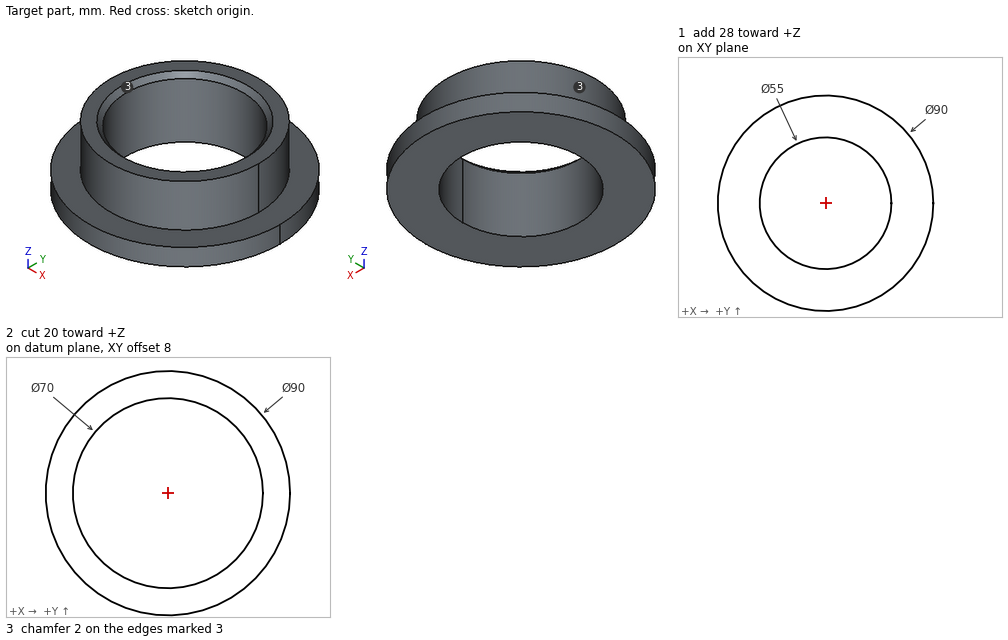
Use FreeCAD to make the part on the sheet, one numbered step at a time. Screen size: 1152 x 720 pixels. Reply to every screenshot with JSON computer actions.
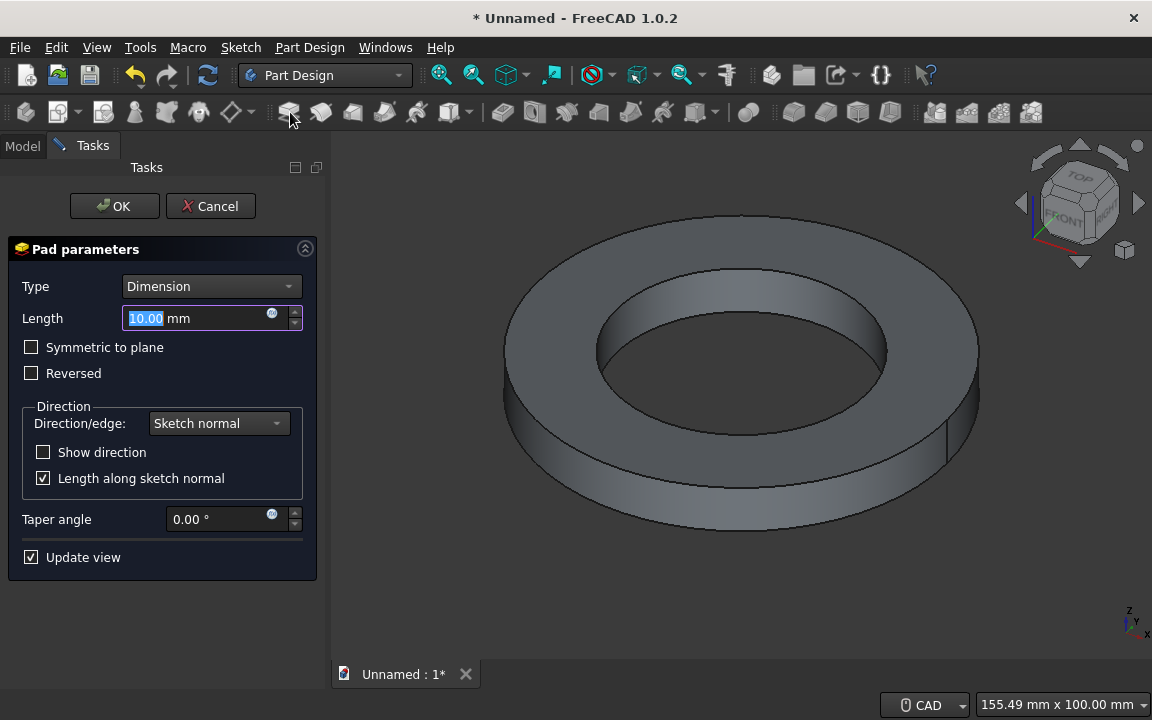
{"action": "type", "text": "28"}
{"action": "key", "text": "Tab"}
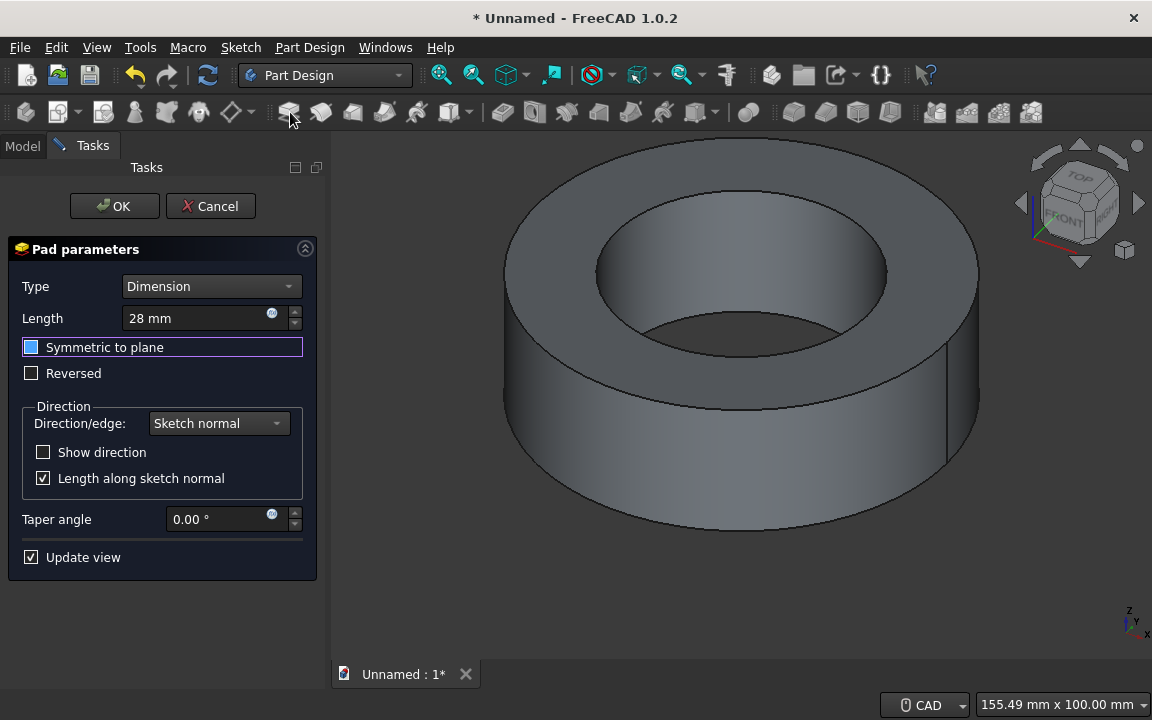
{"action": "left_click", "coordinate": [115, 206]}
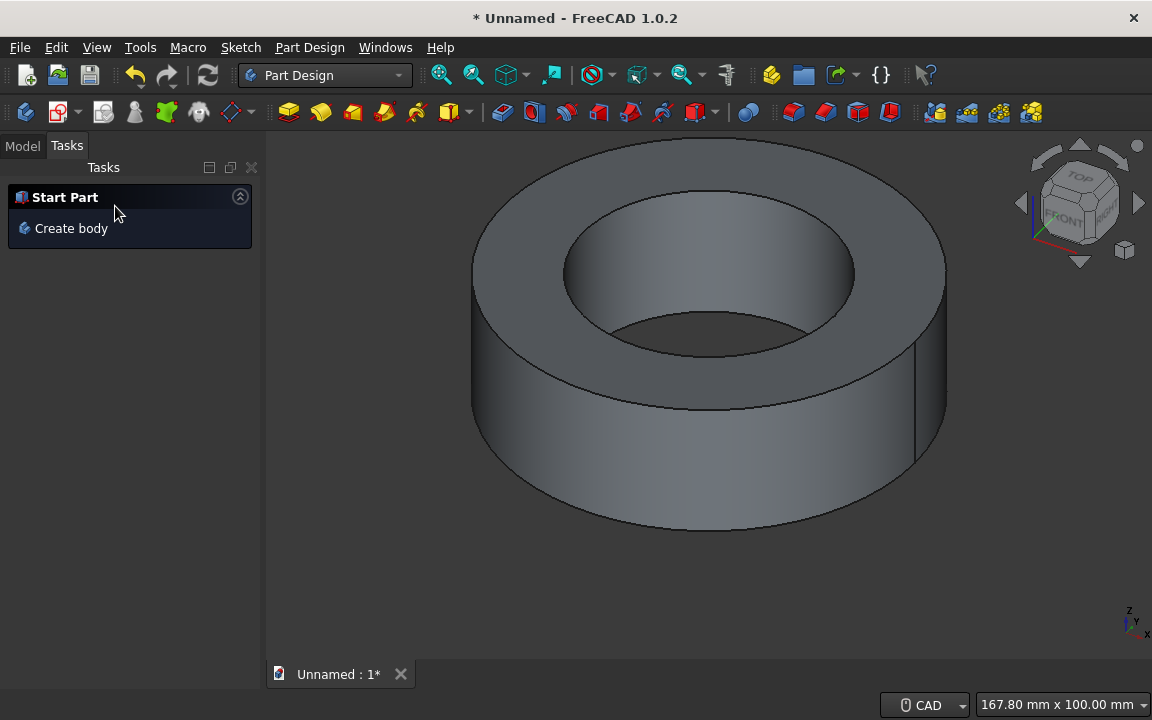
{"action": "left_click", "coordinate": [442, 76]}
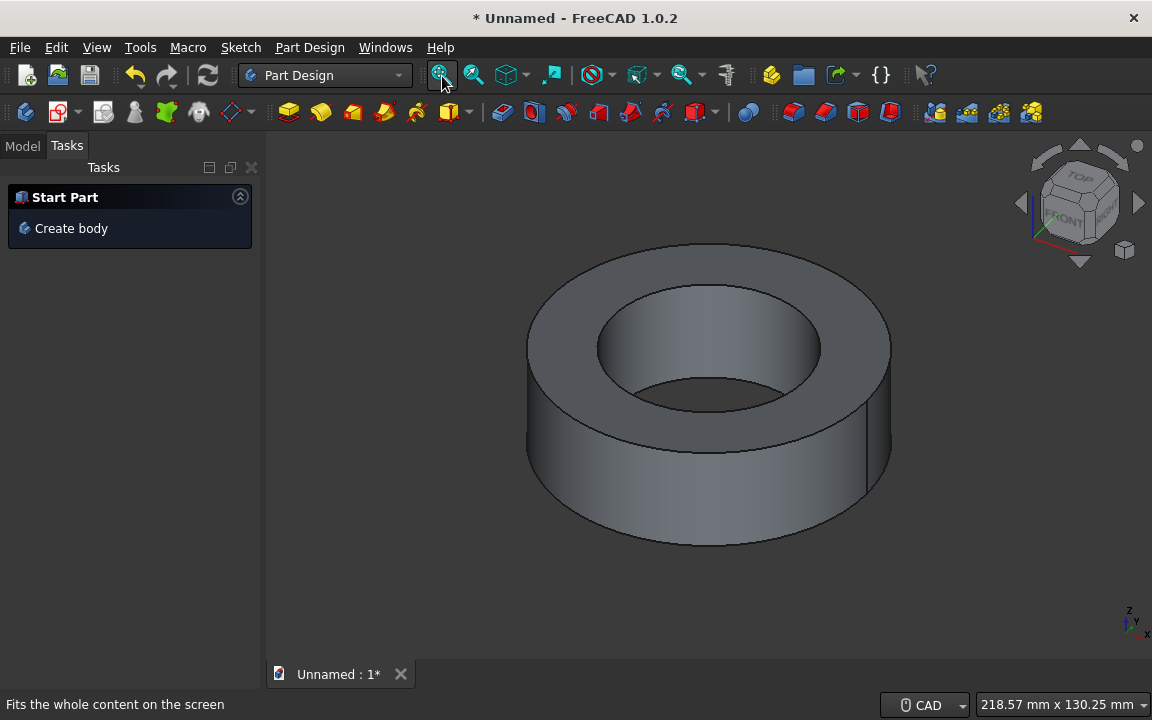
{"action": "left_click", "coordinate": [23, 145]}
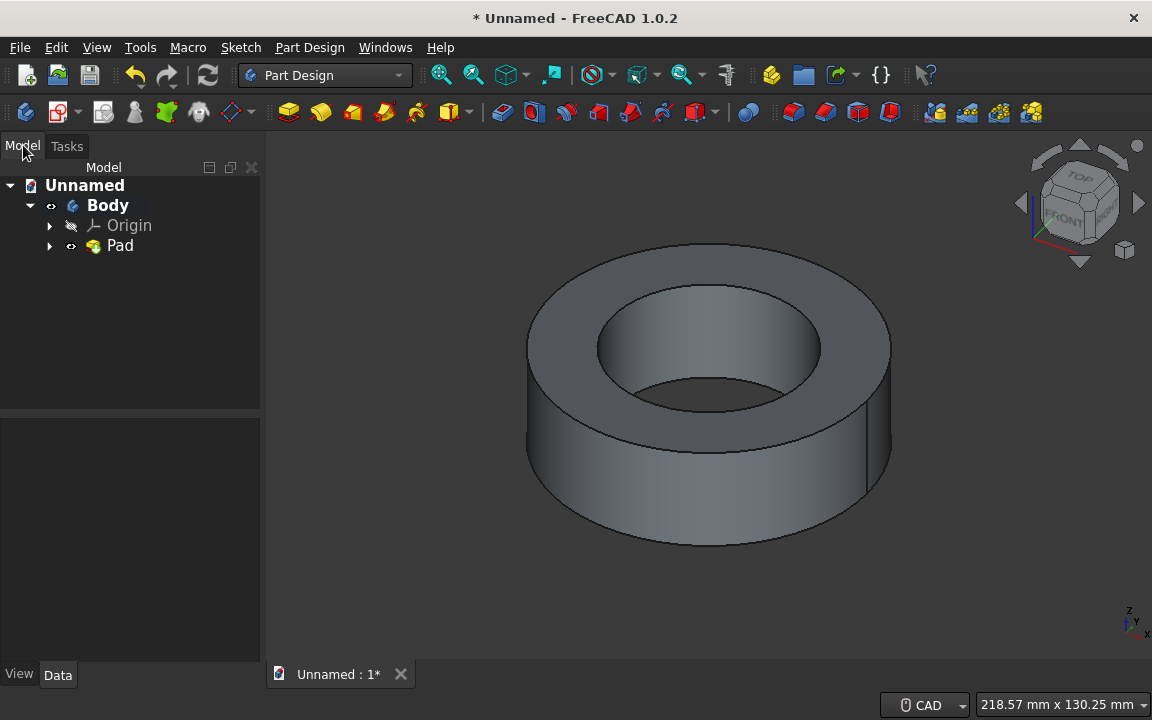
{"action": "left_click", "coordinate": [50, 226]}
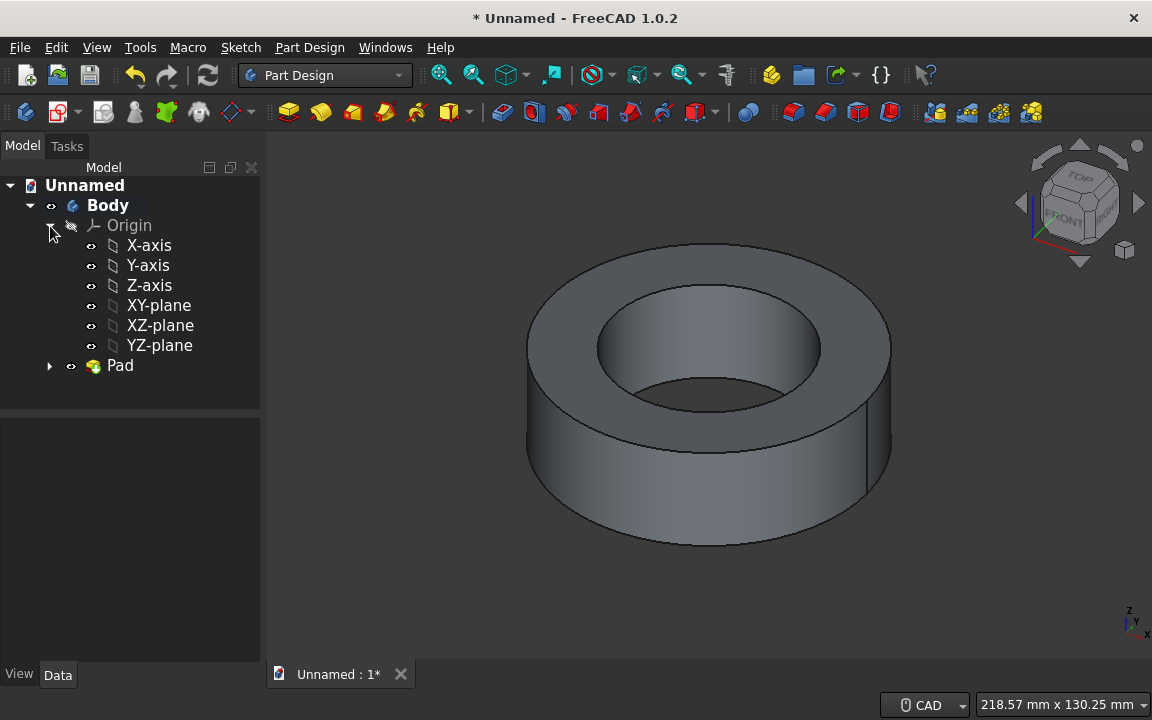
{"action": "left_click", "coordinate": [136, 306]}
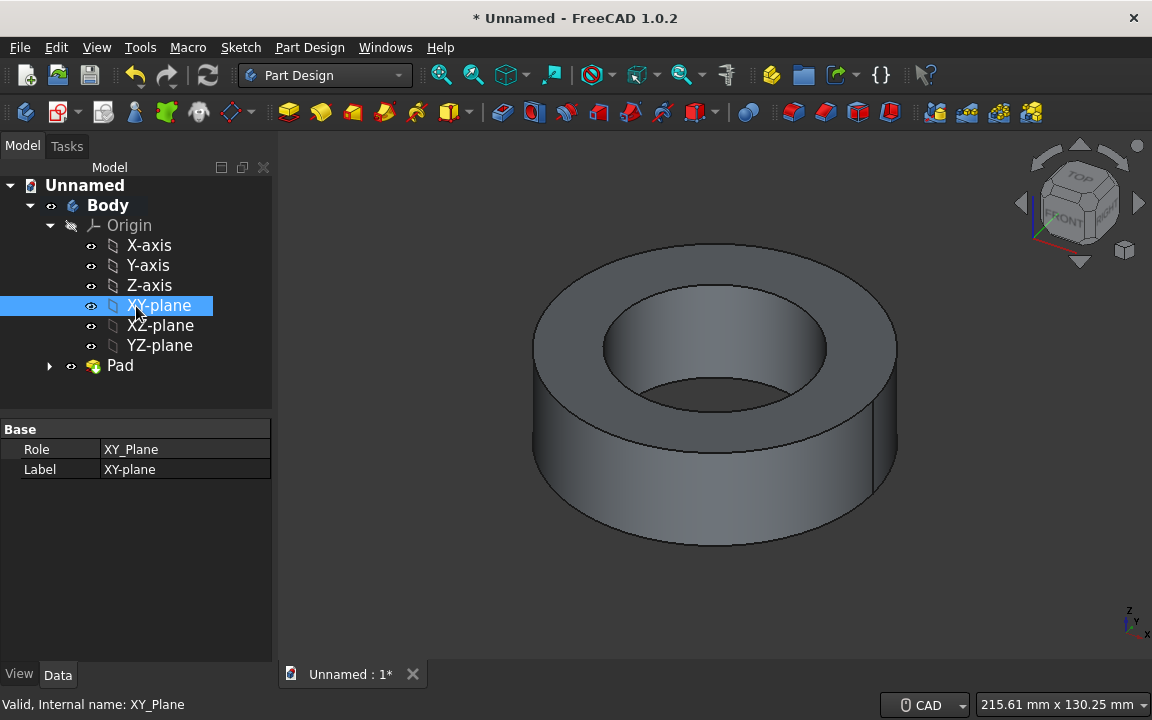
{"action": "left_click", "coordinate": [232, 112]}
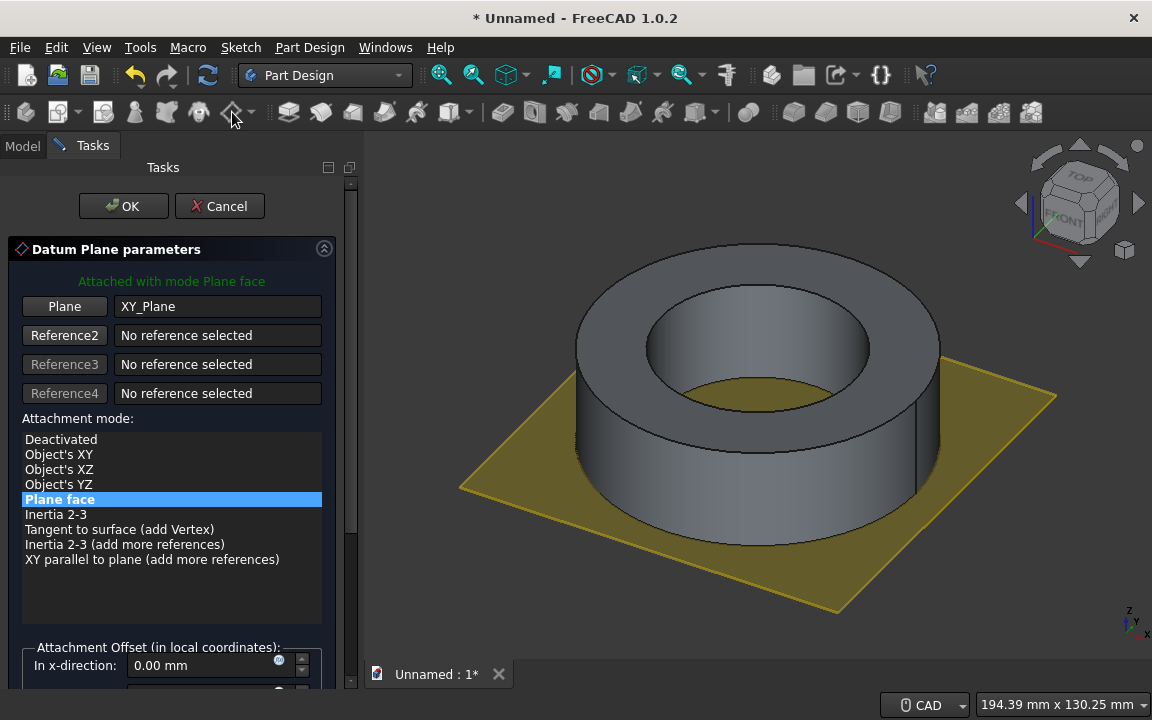
{"action": "scroll", "coordinate": [351, 432], "scroll_direction": "down", "scroll_amount": 2}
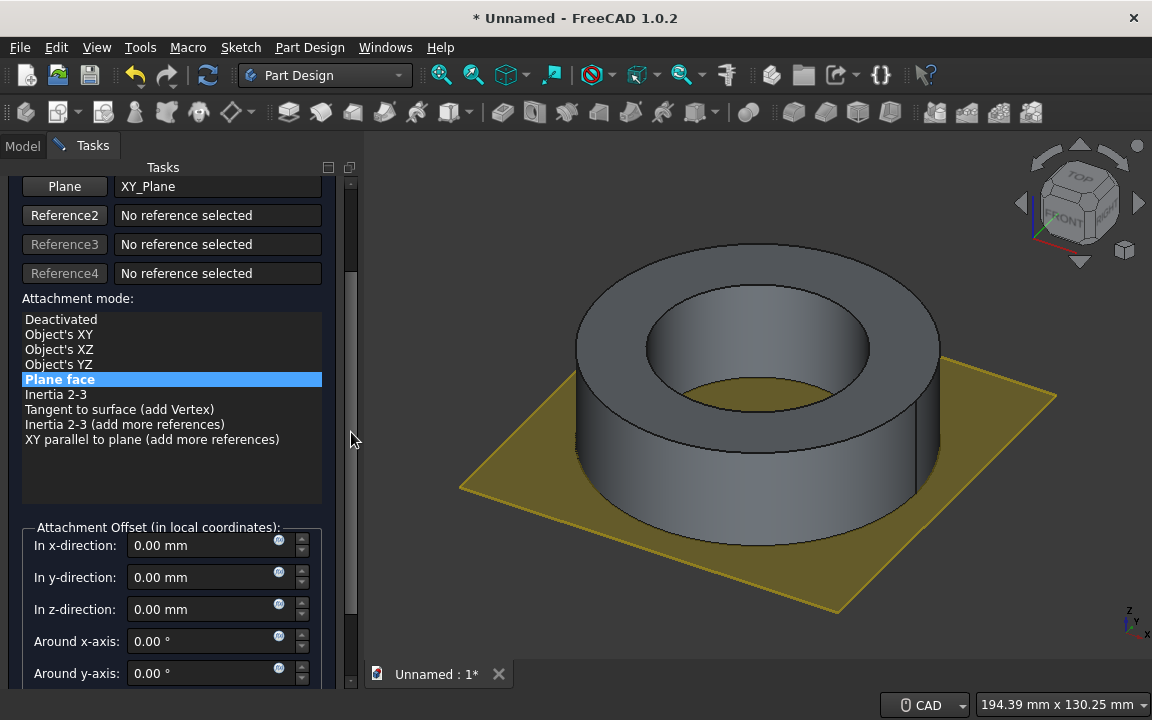
{"action": "triple_click", "coordinate": [210, 609]}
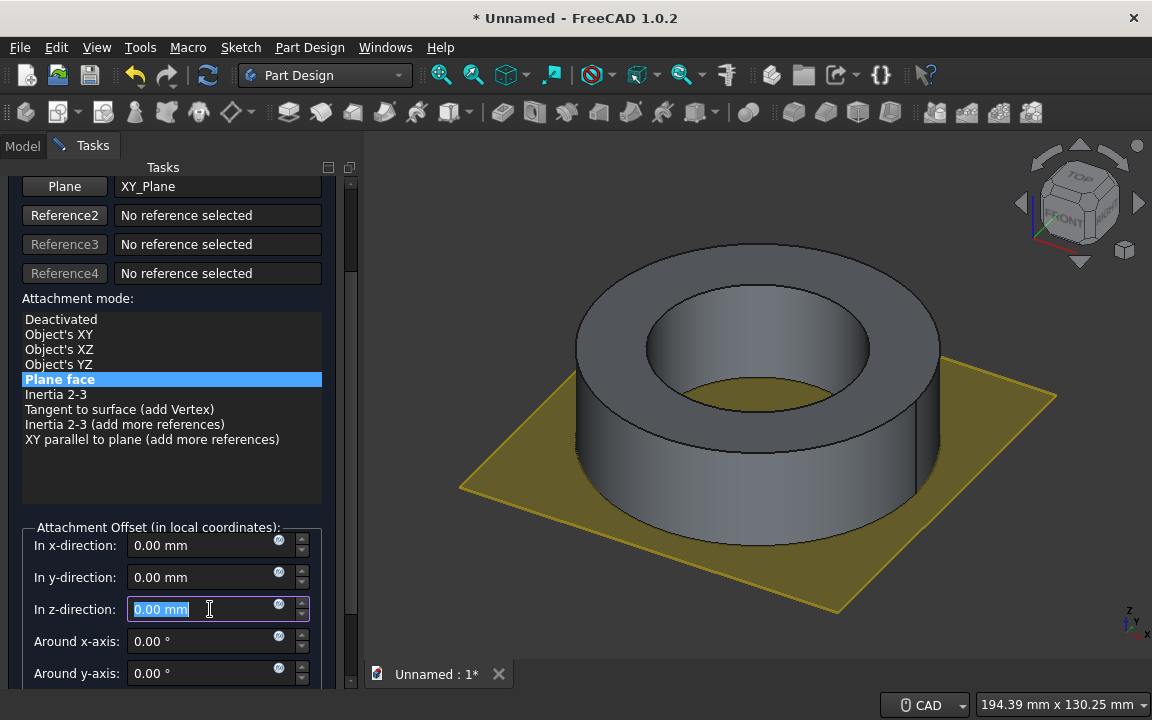
{"action": "type", "text": "8"}
{"action": "key", "text": "Tab"}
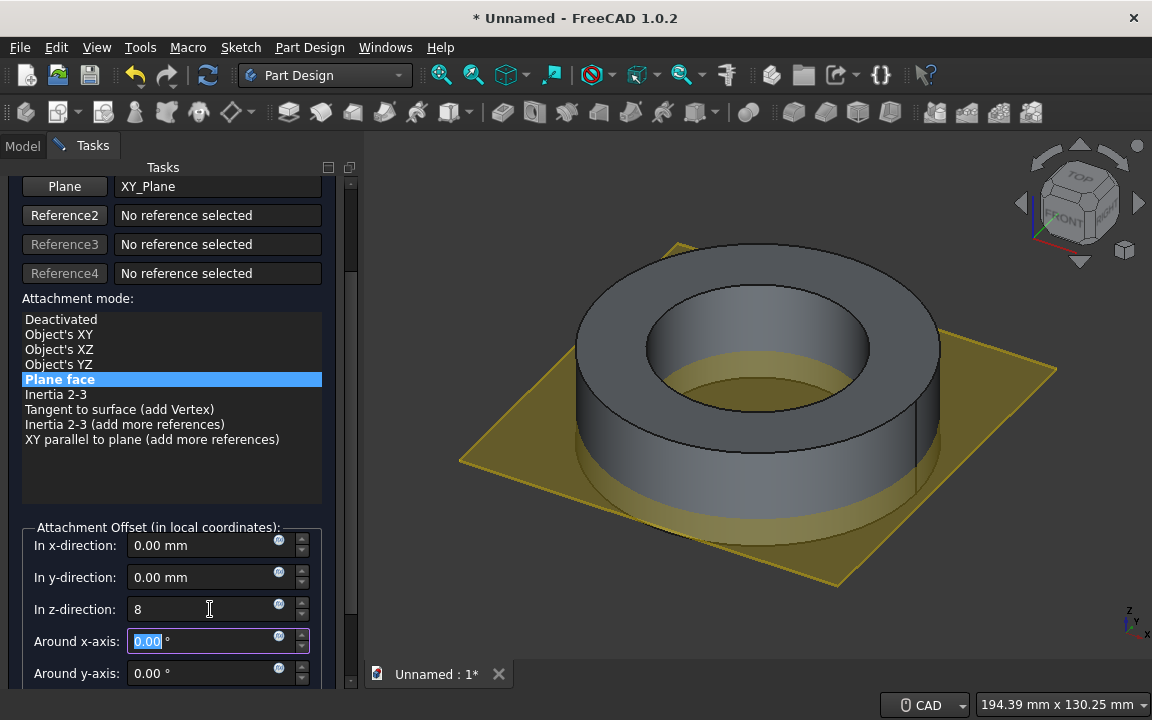
{"action": "scroll", "coordinate": [351, 432], "scroll_direction": "up", "scroll_amount": 3}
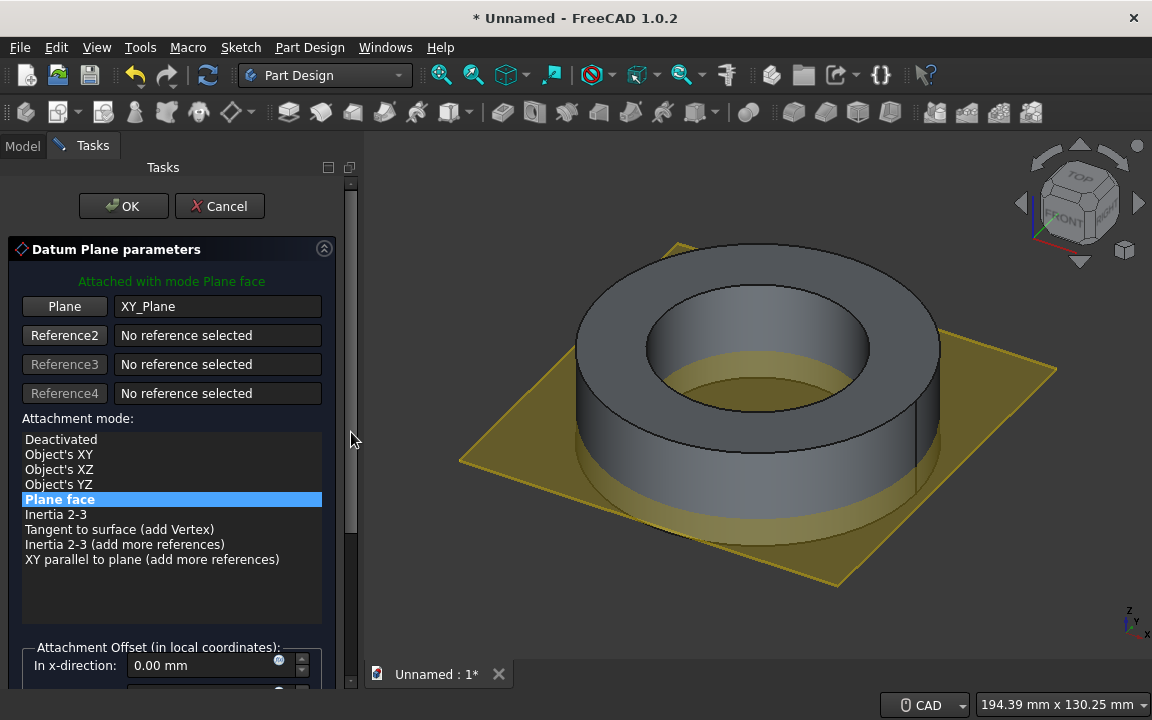
{"action": "left_click", "coordinate": [124, 206]}